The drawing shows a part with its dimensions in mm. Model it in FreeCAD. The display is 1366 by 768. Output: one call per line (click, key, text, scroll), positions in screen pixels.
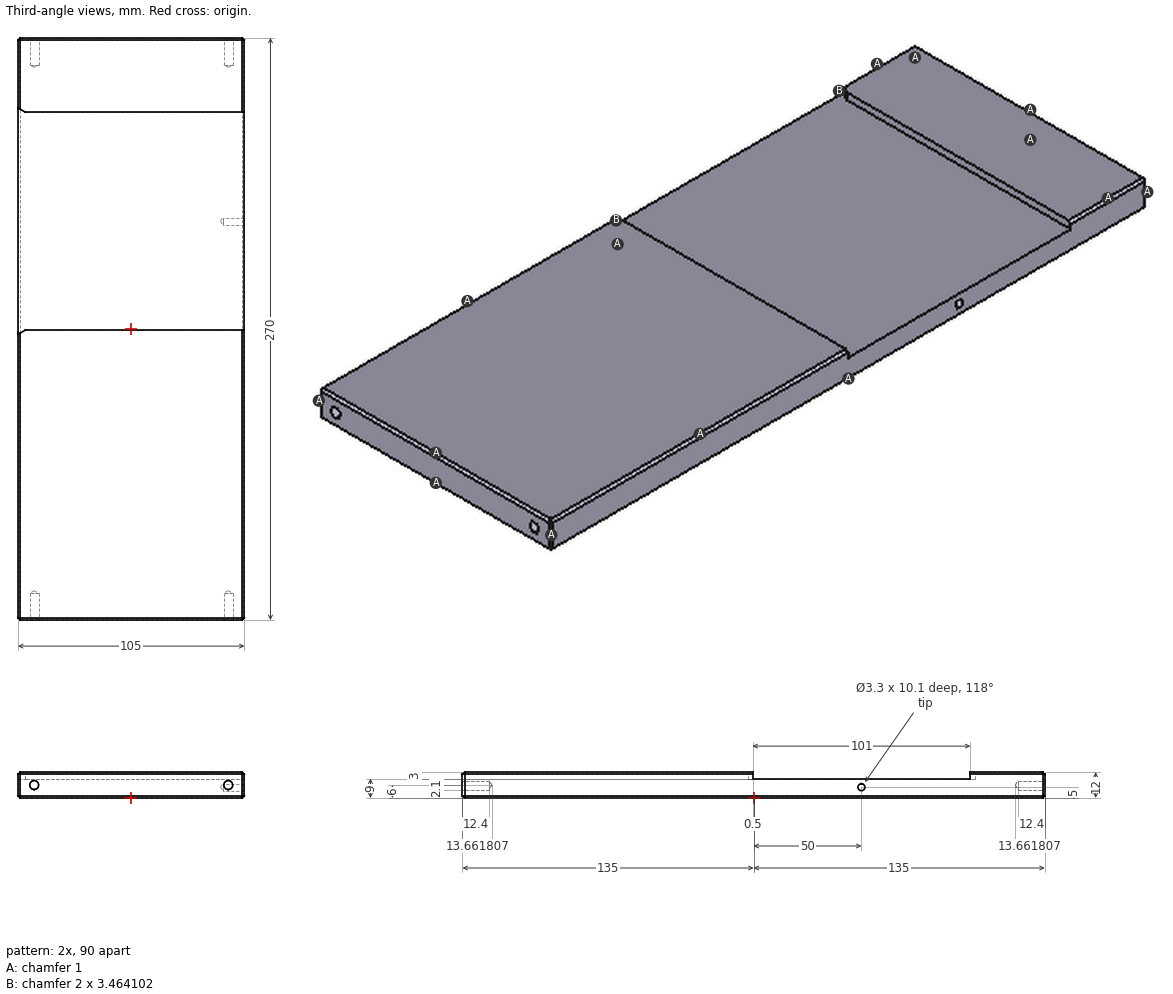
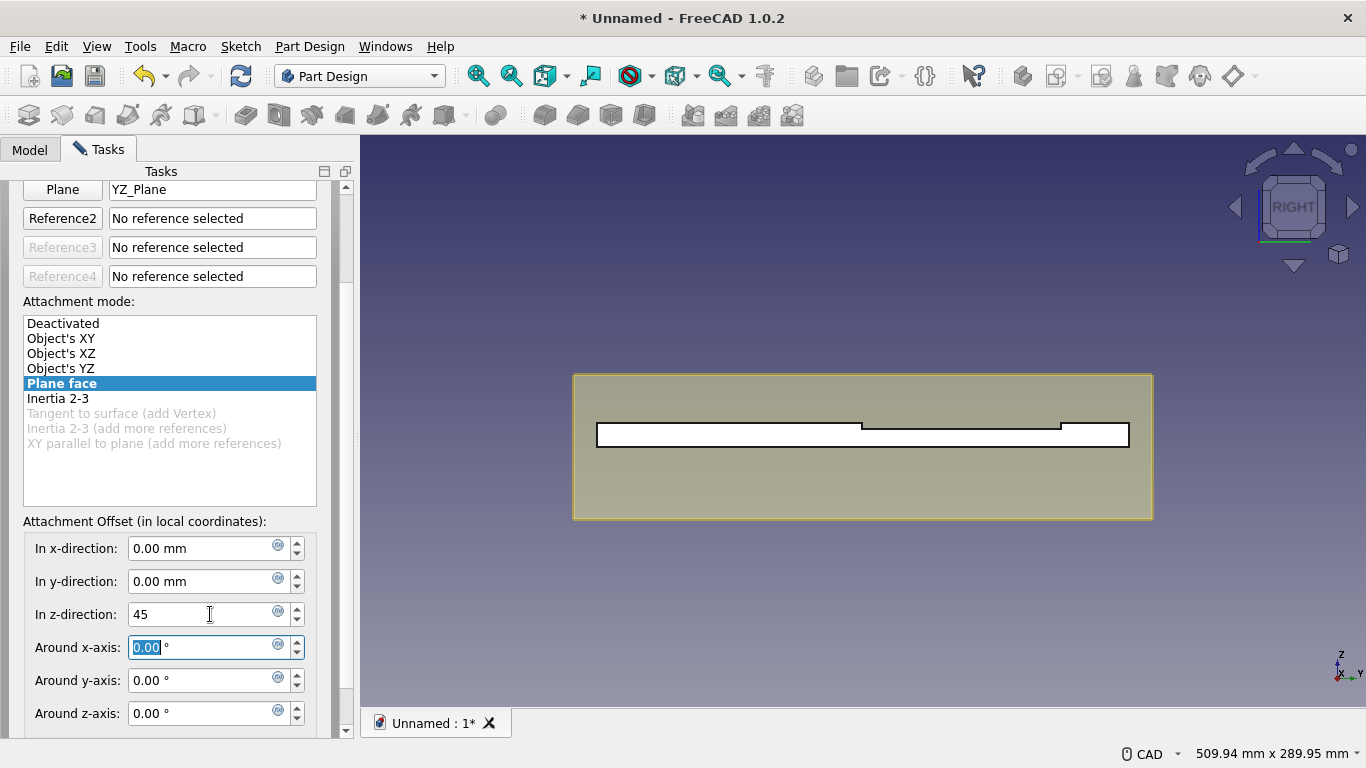
scroll(346, 460, up, 3)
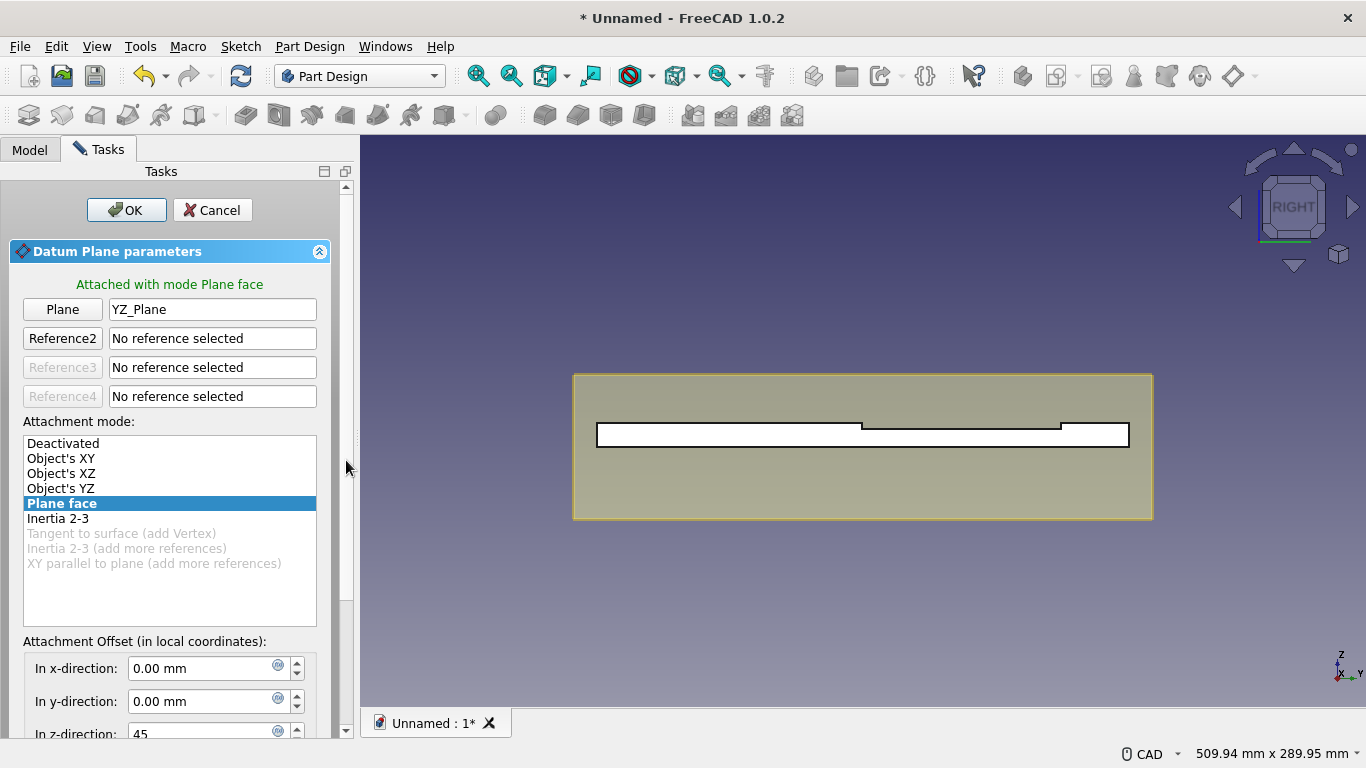
click(127, 210)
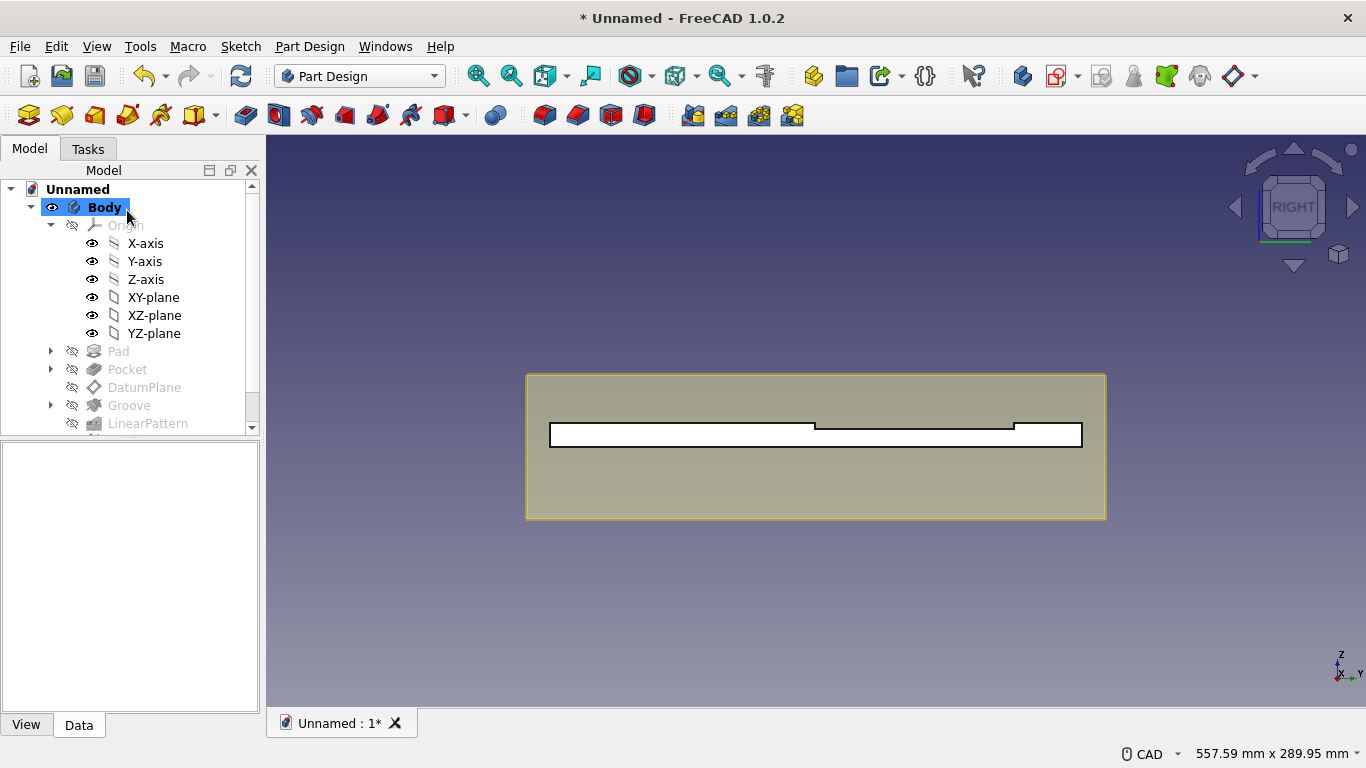
scroll(101, 311, down, 3)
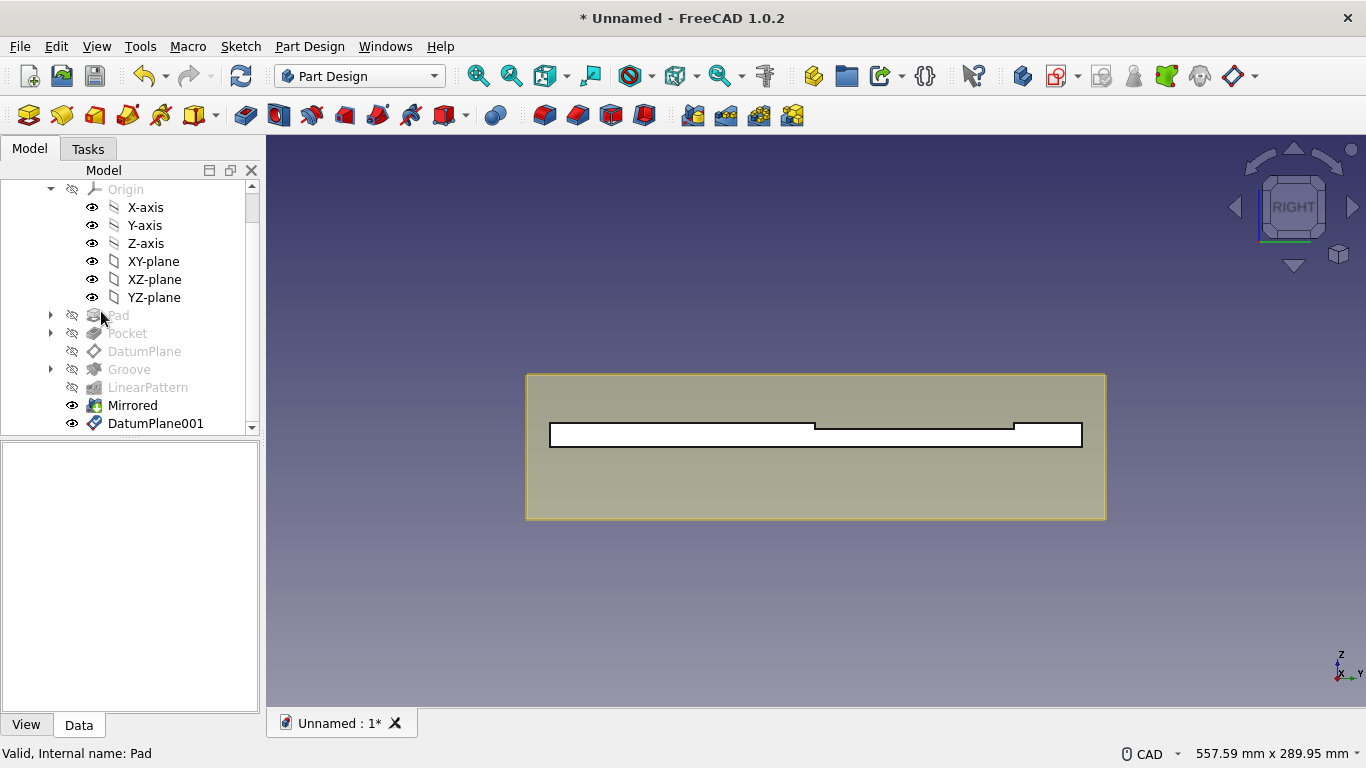
click(117, 423)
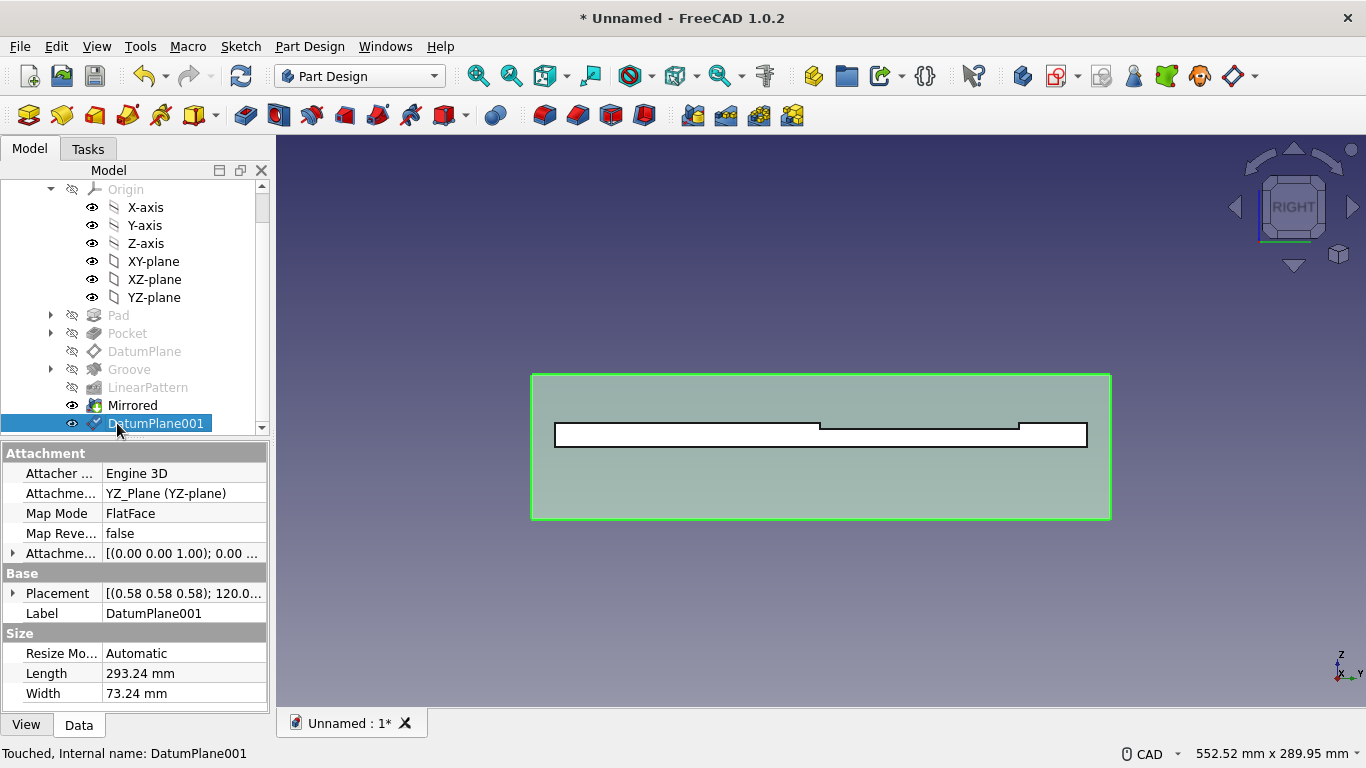
click(1056, 76)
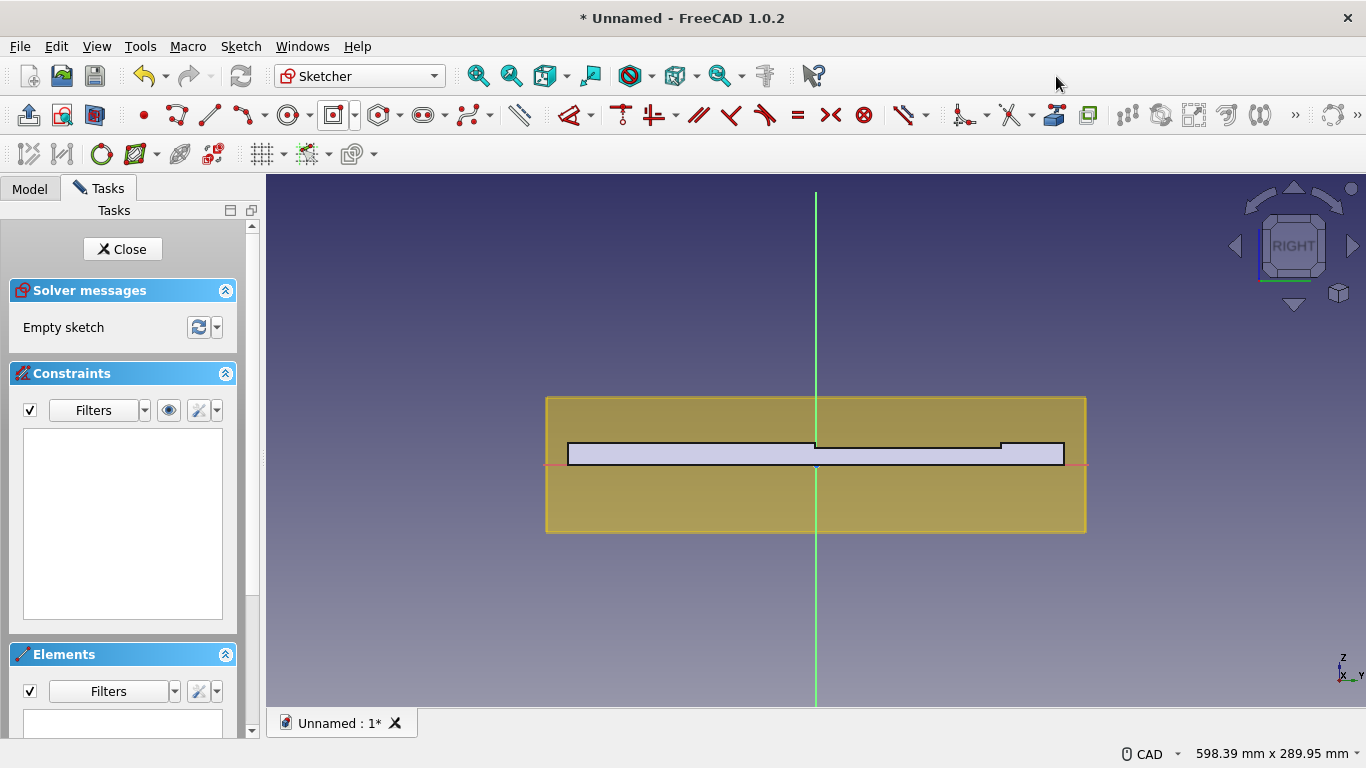
click(95, 116)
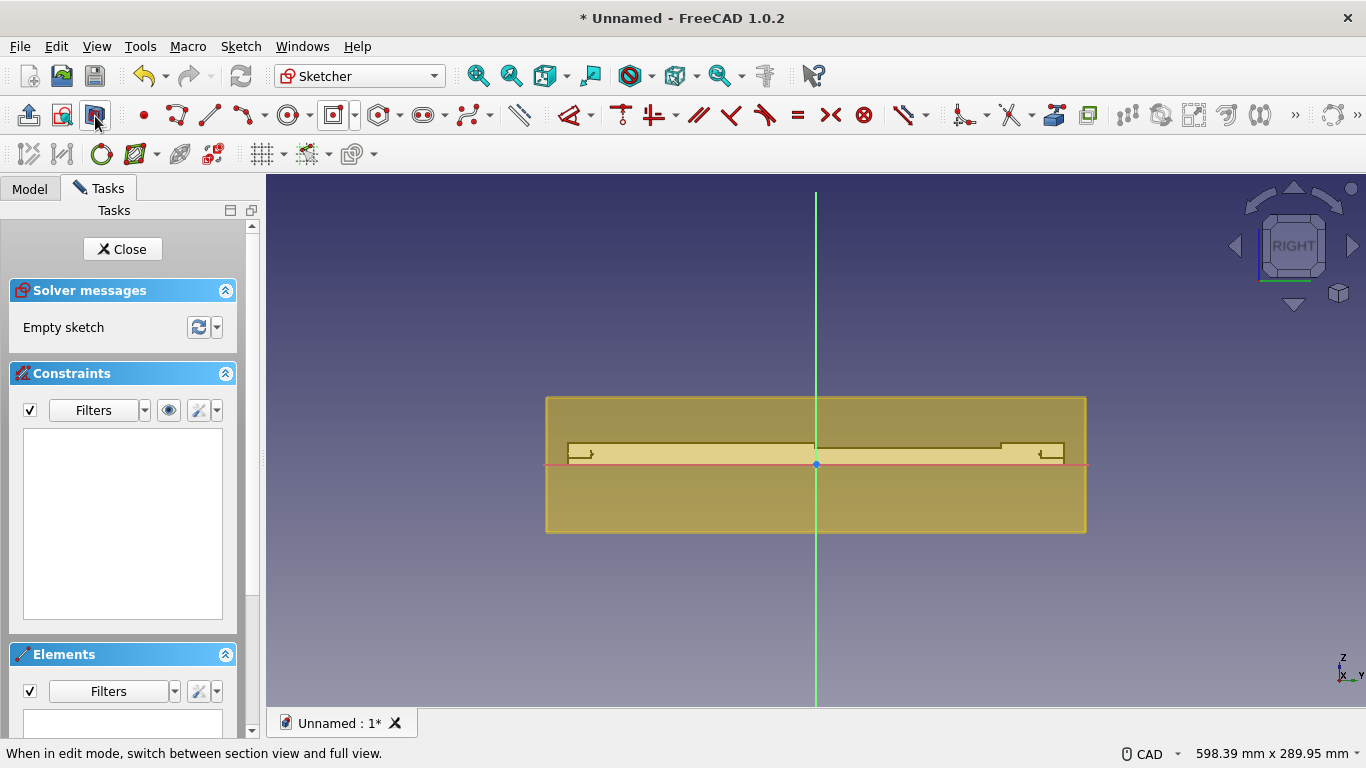
scroll(1073, 457, up, 15)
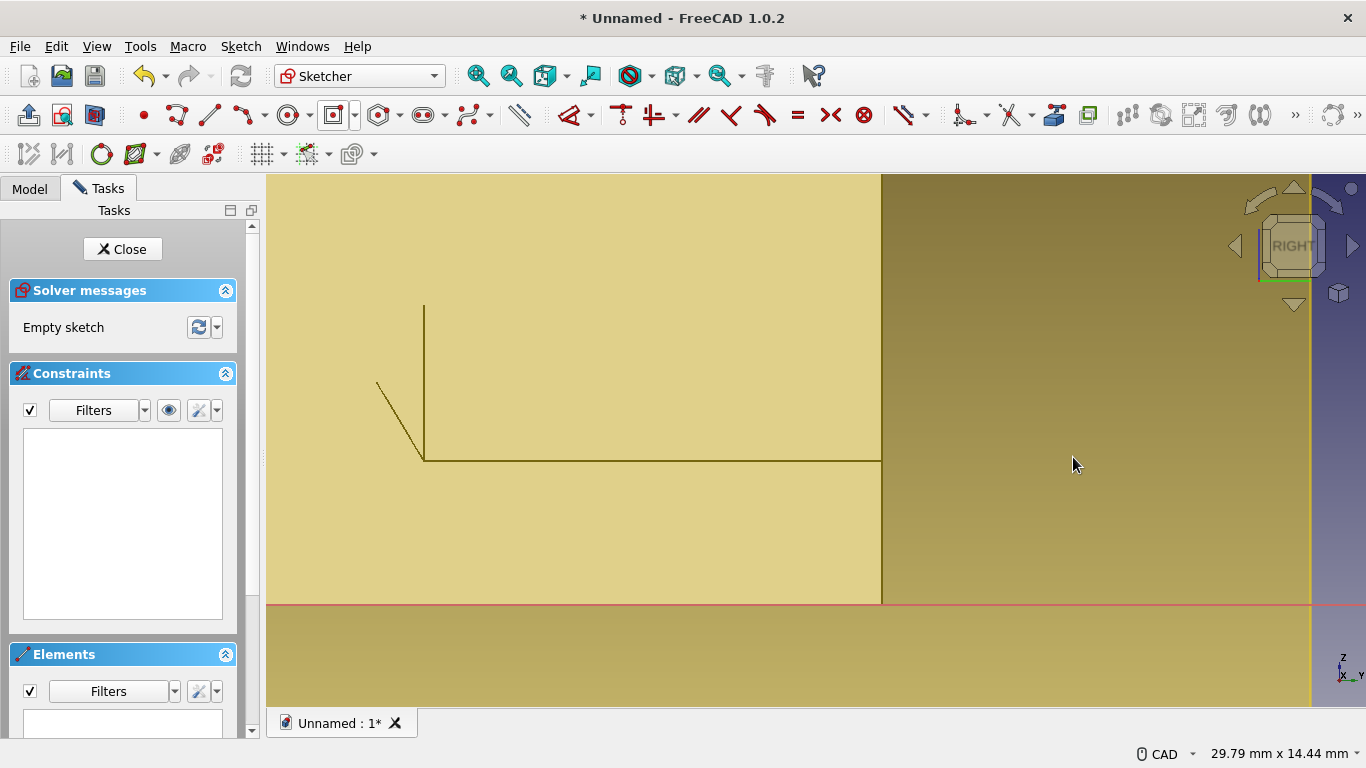
click(177, 116)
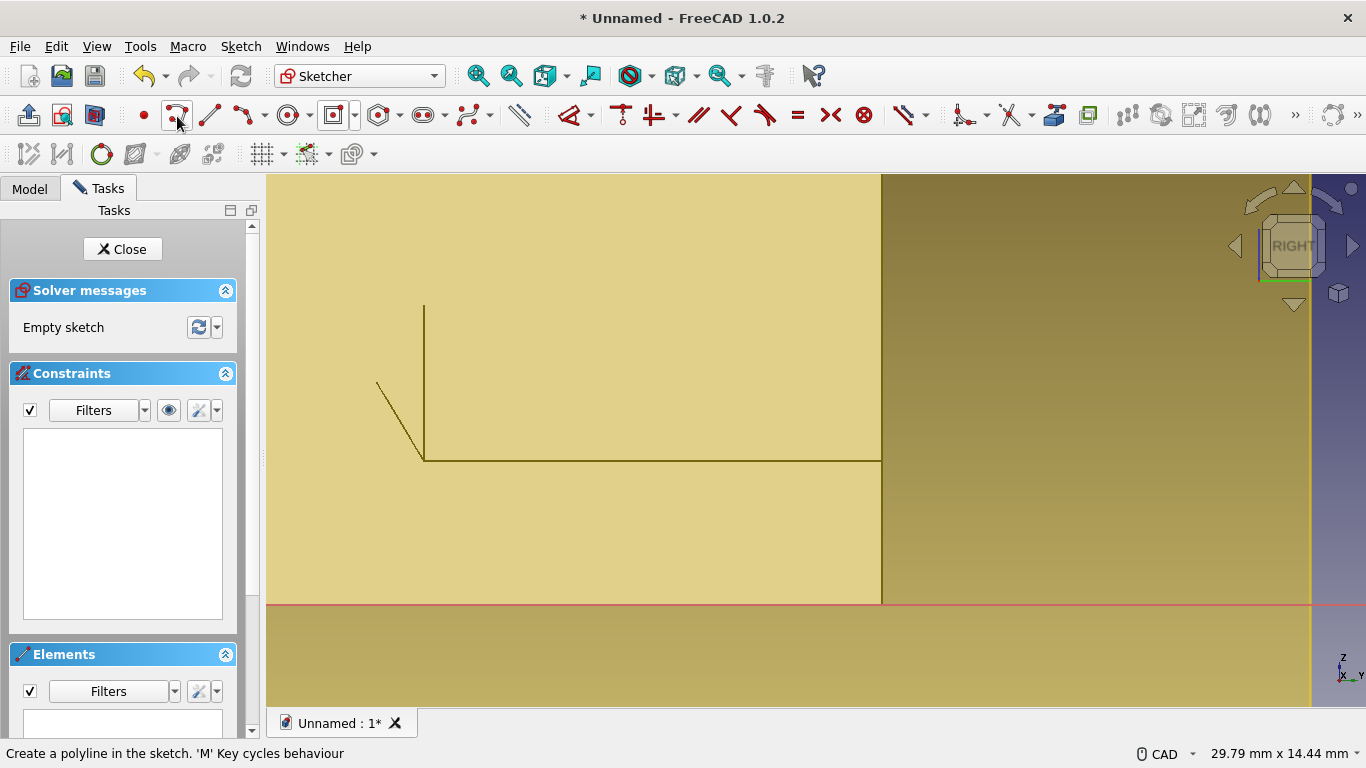
click(377, 383)
click(424, 461)
click(882, 461)
click(882, 383)
click(377, 384)